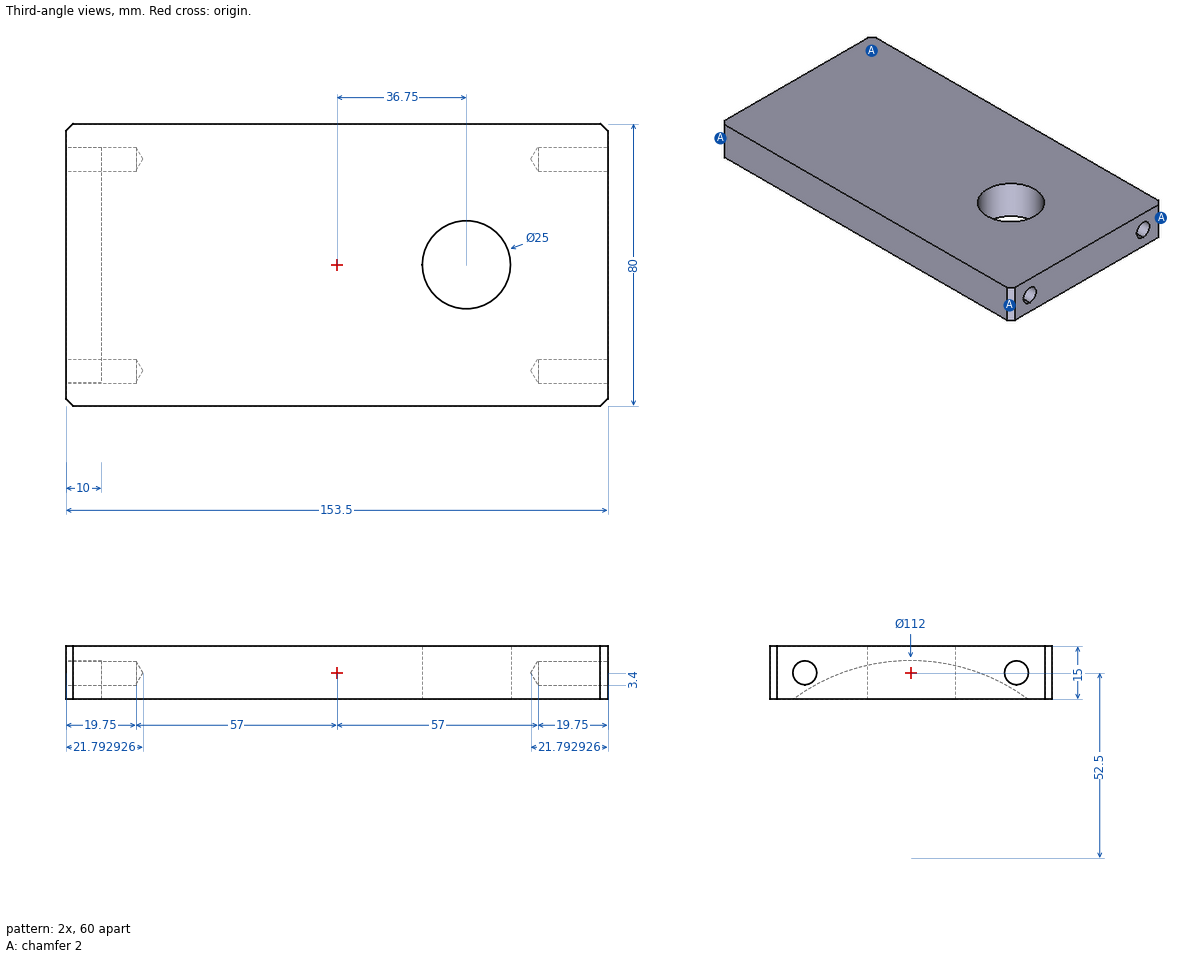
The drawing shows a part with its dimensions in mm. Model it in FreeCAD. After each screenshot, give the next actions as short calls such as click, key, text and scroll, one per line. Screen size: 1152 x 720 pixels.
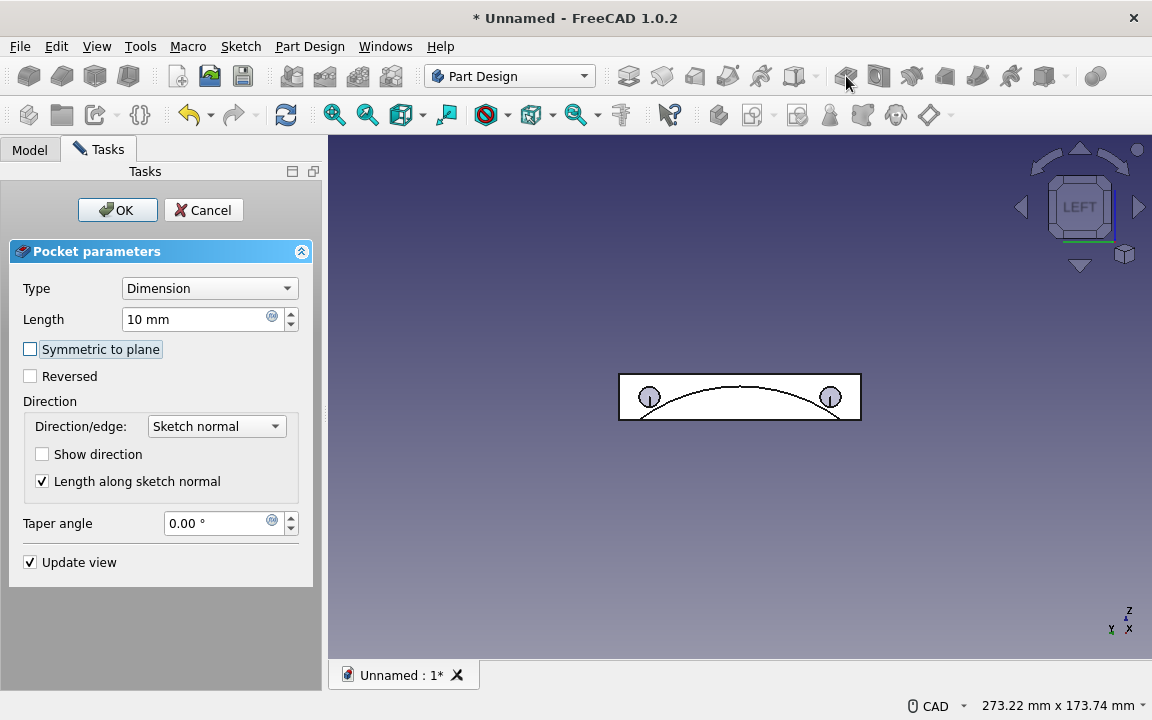
click(118, 210)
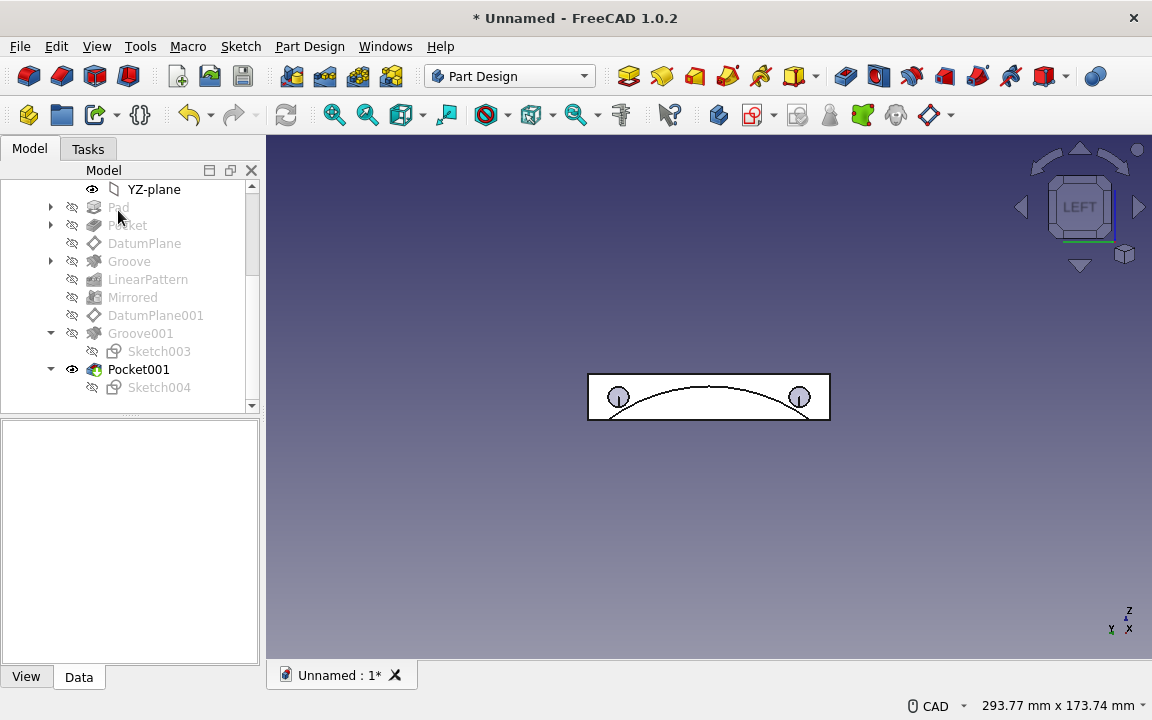
click(335, 116)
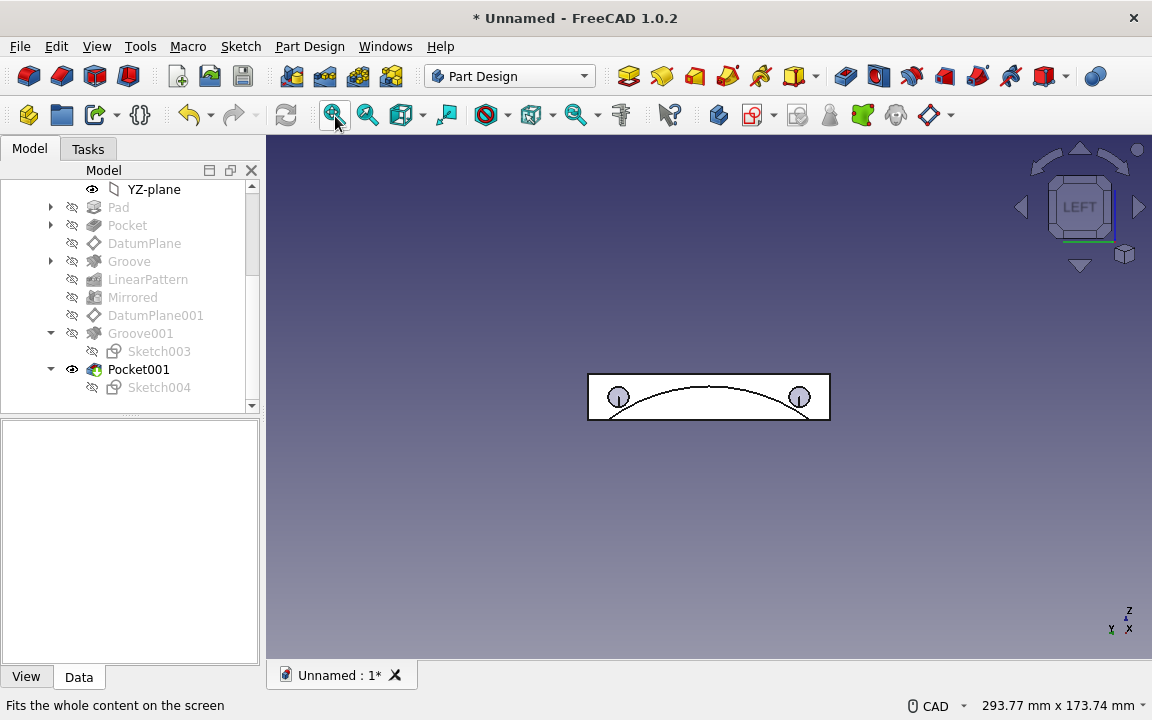
click(830, 396)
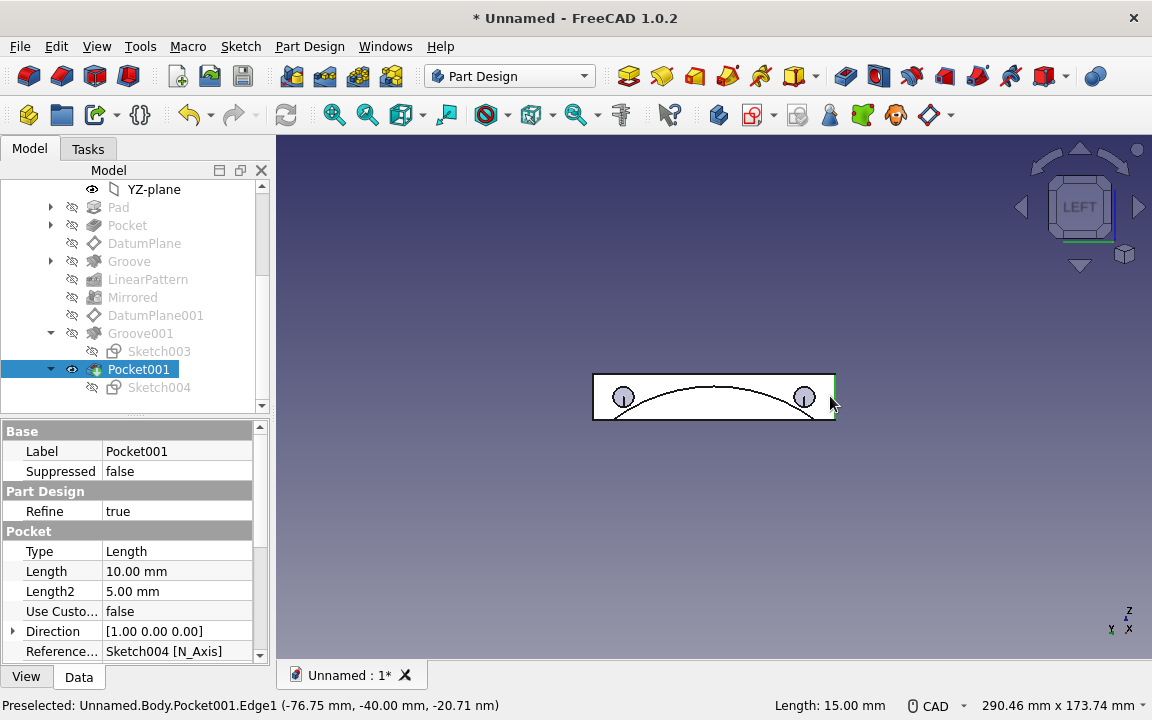
click(593, 396, ctrl)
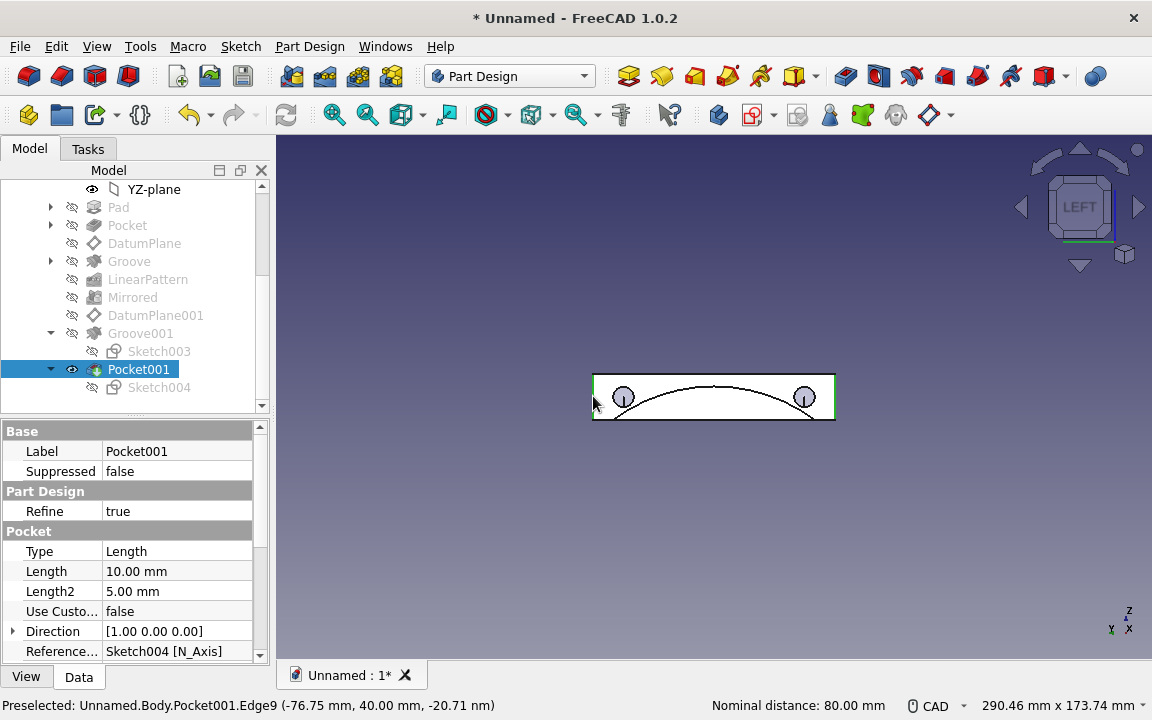
key(0)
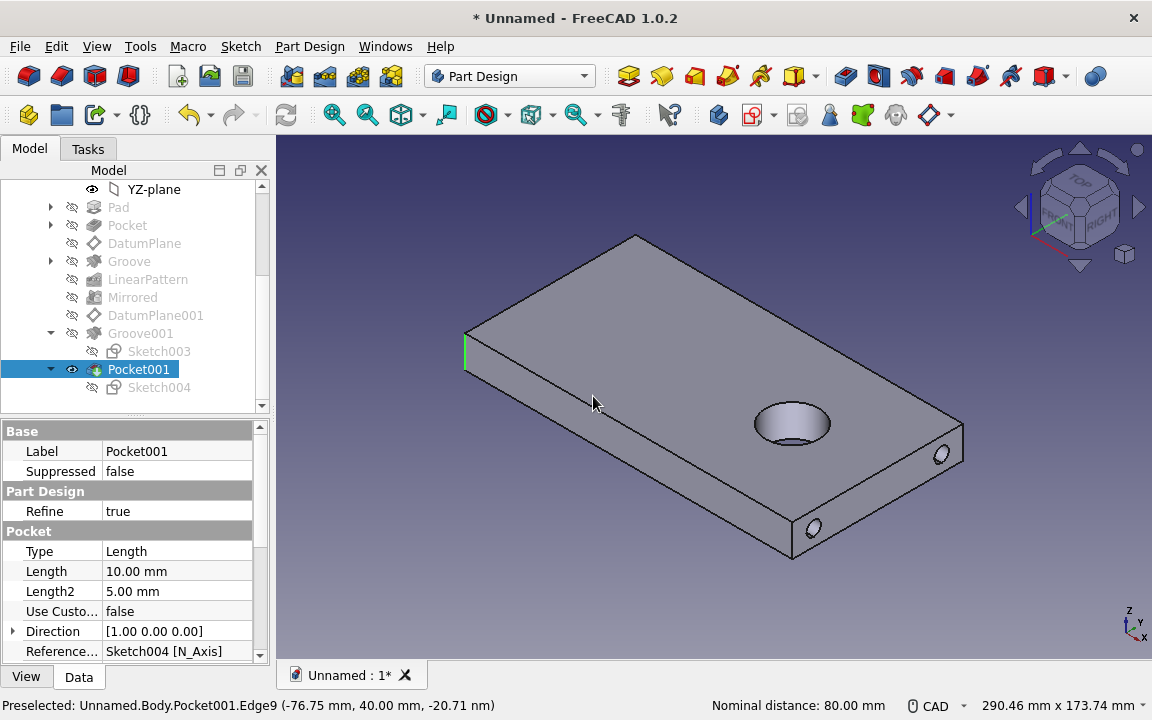
click(792, 540, ctrl)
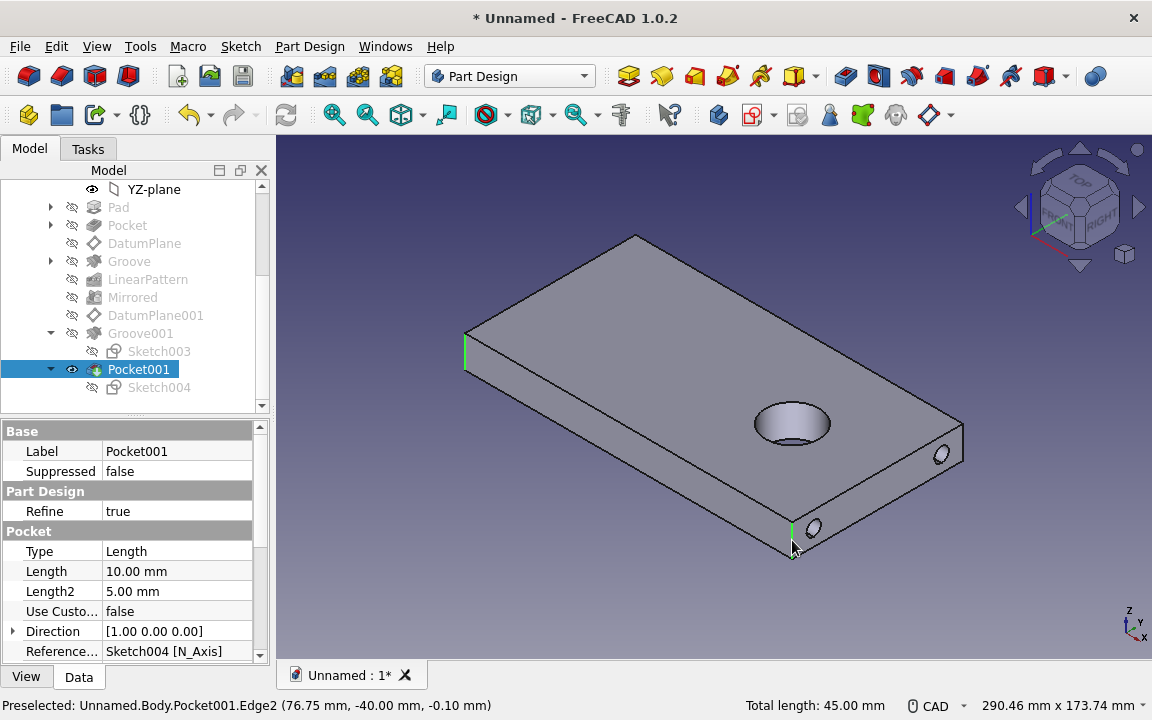
key(2)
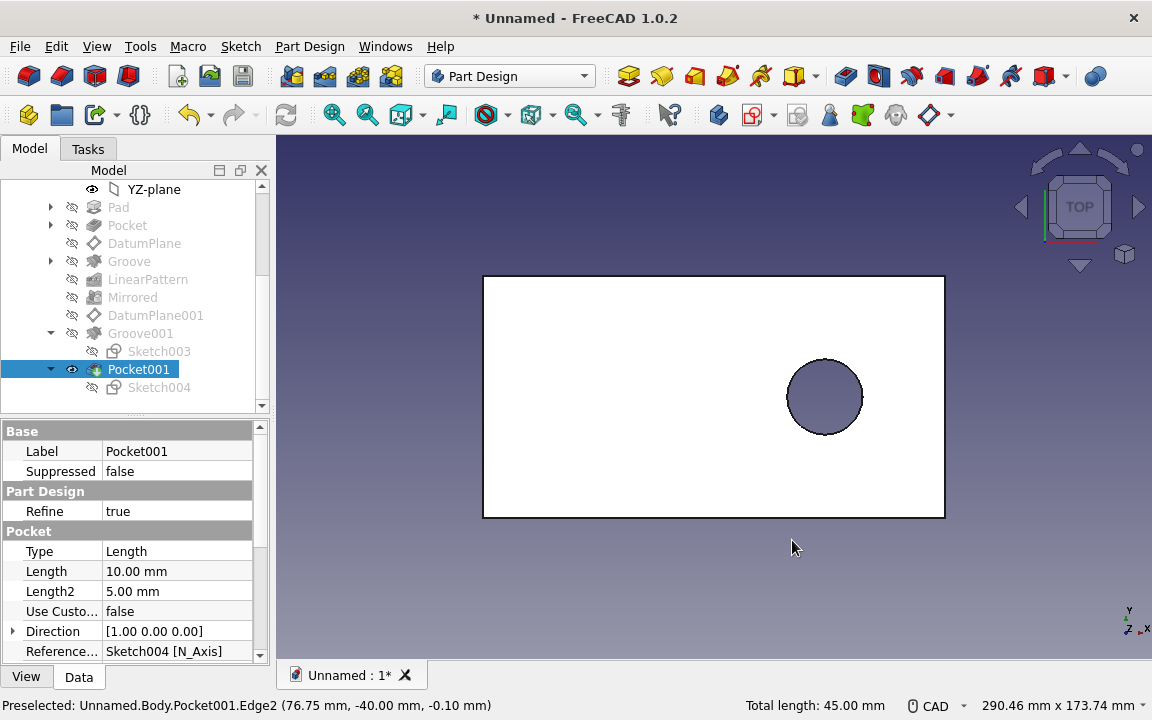
key(1)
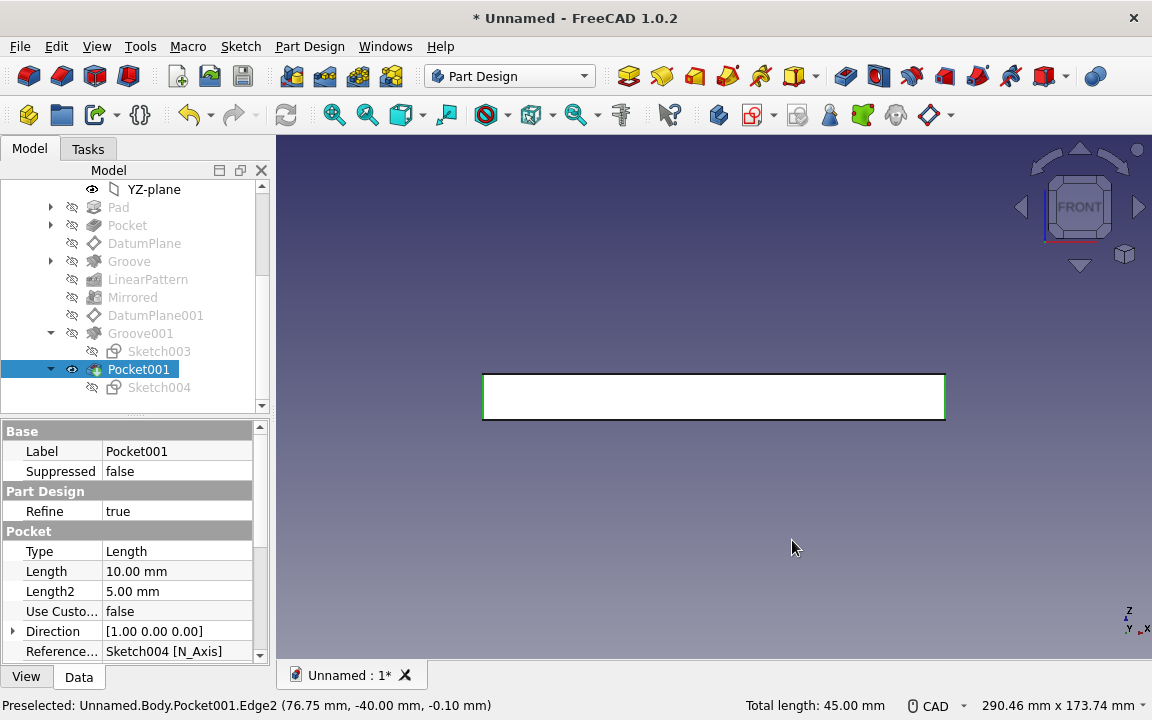
key(3)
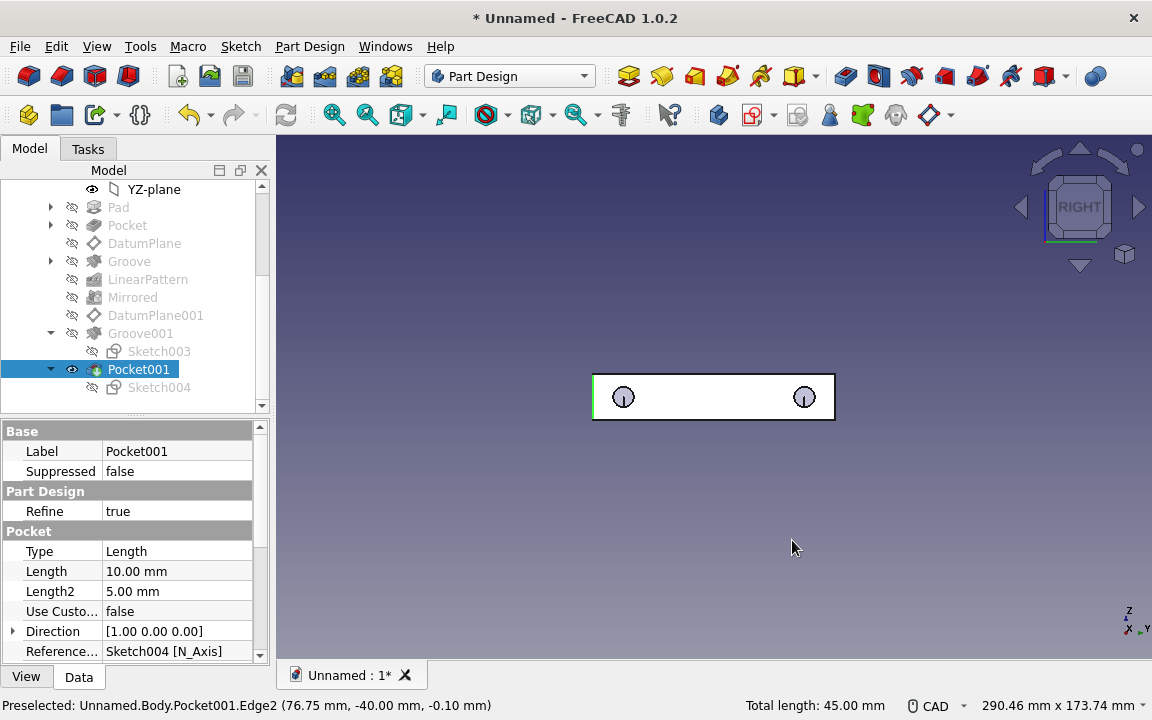
click(335, 116)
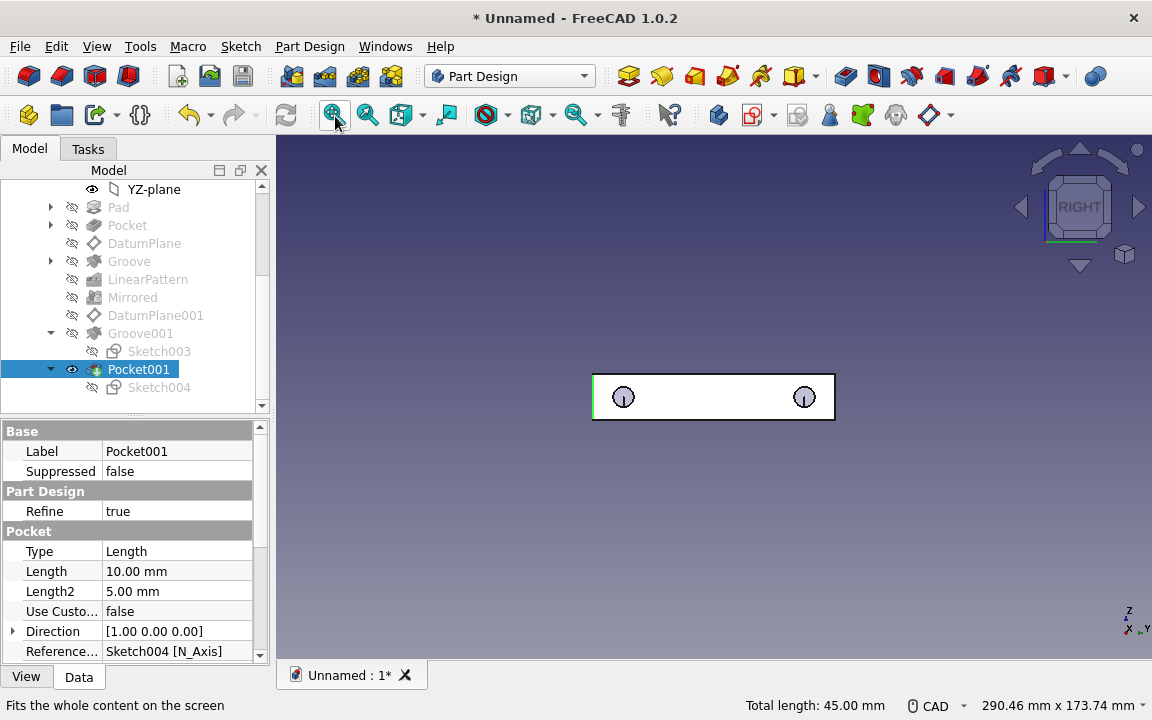
click(835, 396, ctrl)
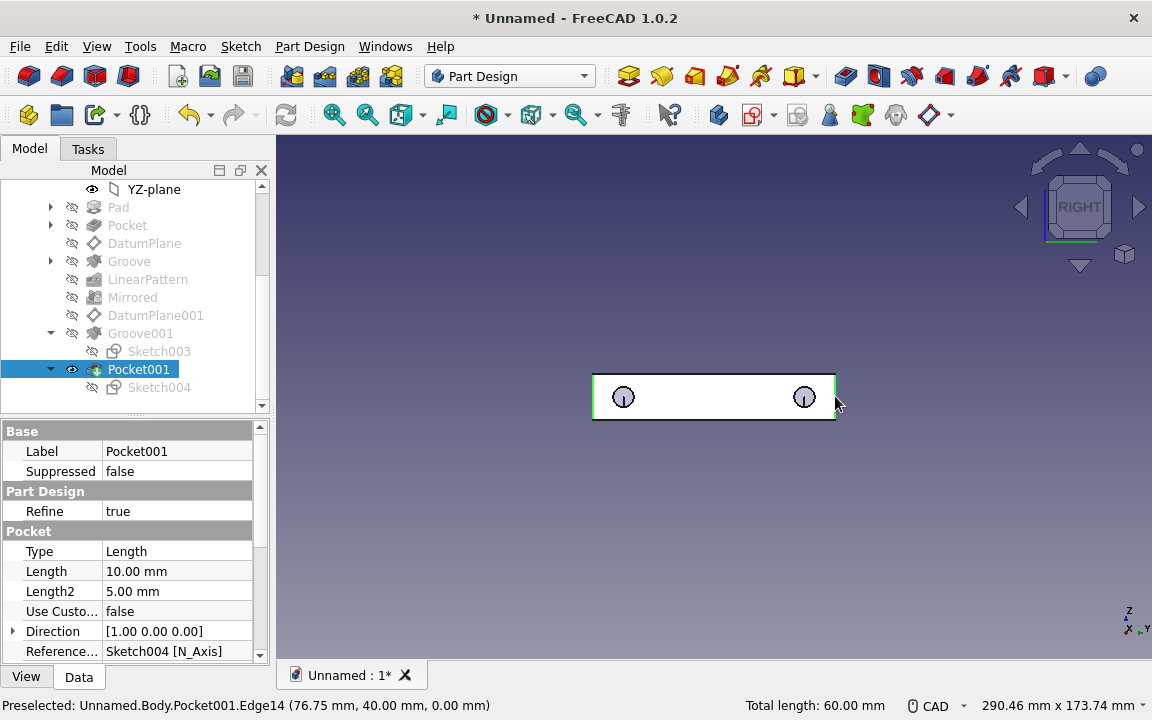
click(62, 76)